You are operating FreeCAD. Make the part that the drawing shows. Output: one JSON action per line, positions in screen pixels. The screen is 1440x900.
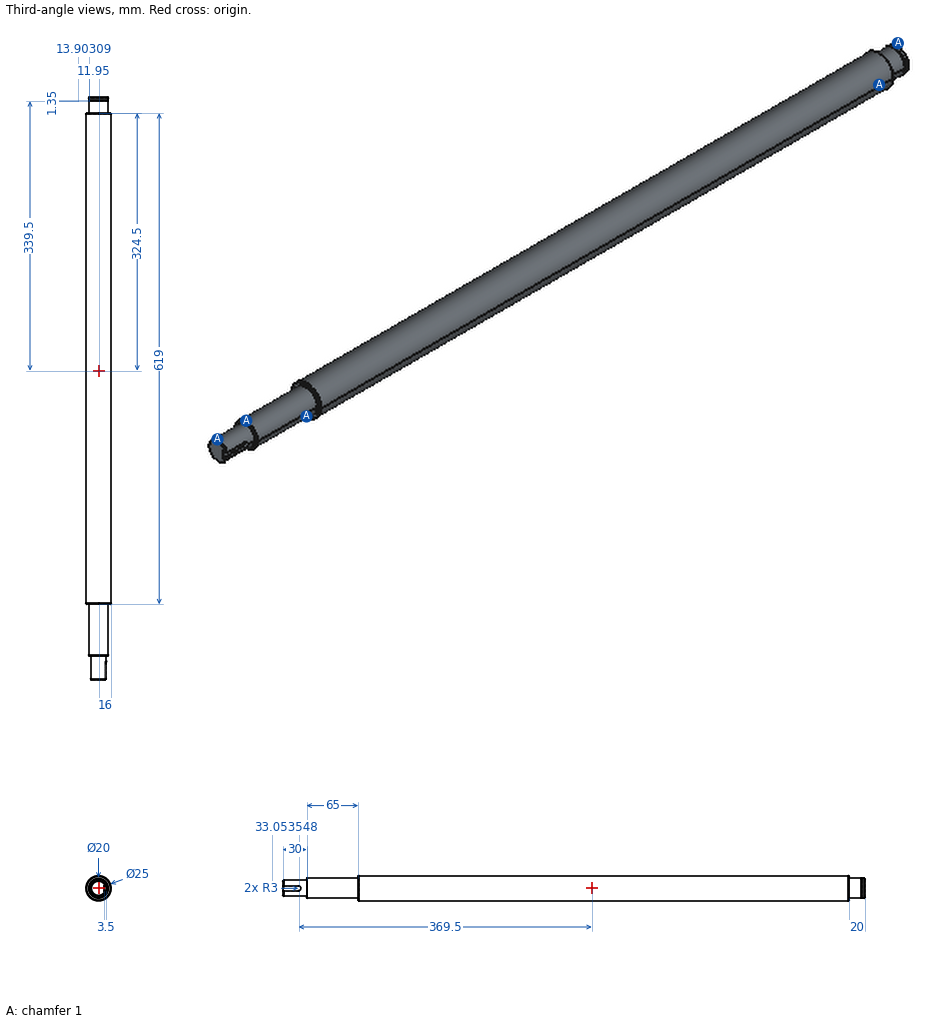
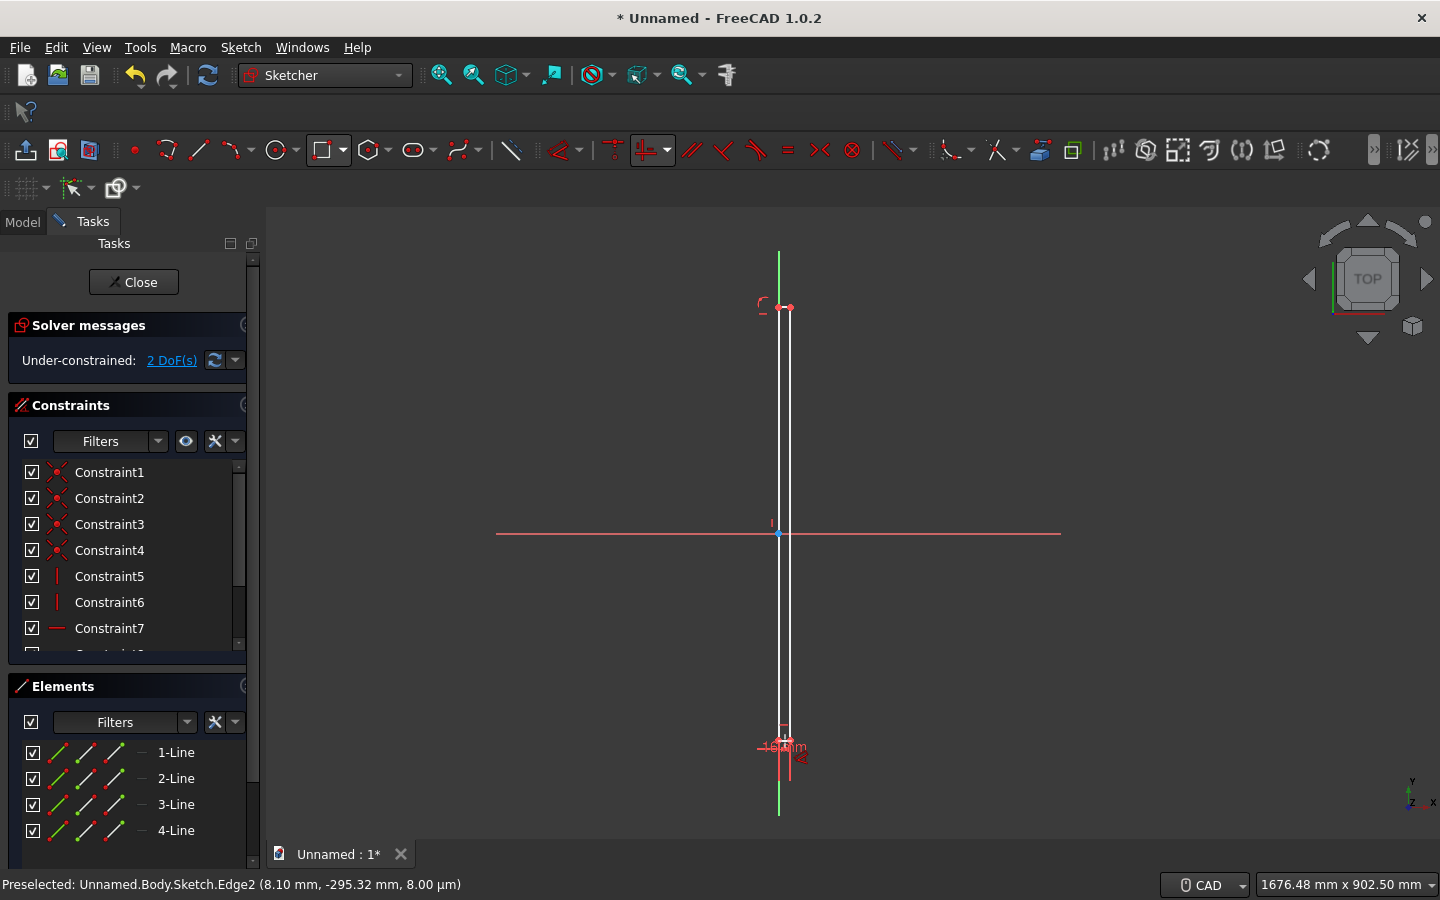
{"action": "scroll", "coordinate": [779, 654], "scroll_direction": "up", "scroll_amount": 2}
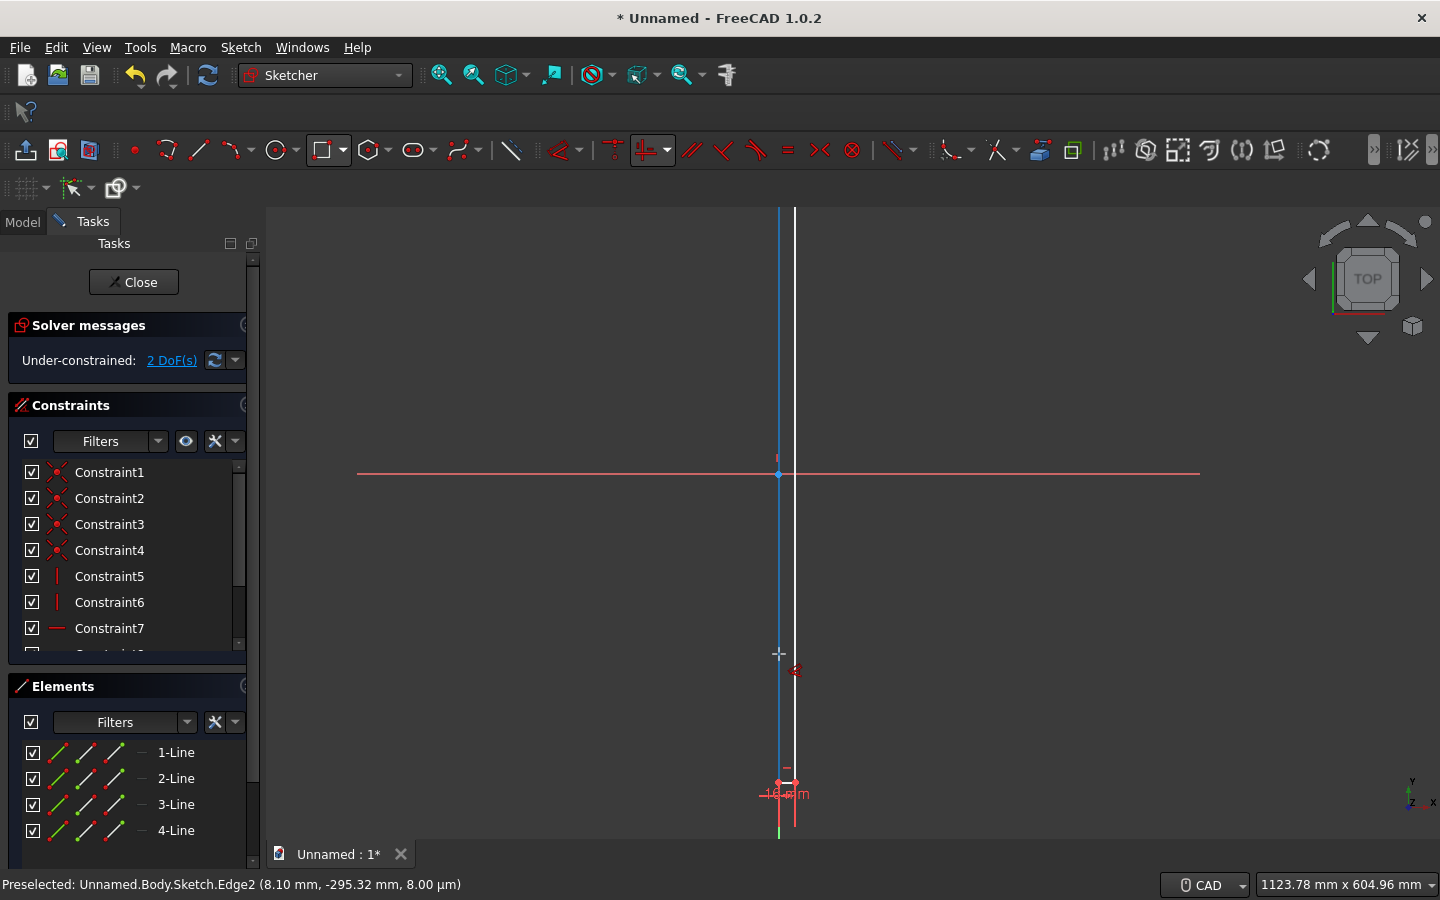
{"action": "left_click", "coordinate": [779, 654]}
{"action": "left_click", "coordinate": [745, 509]}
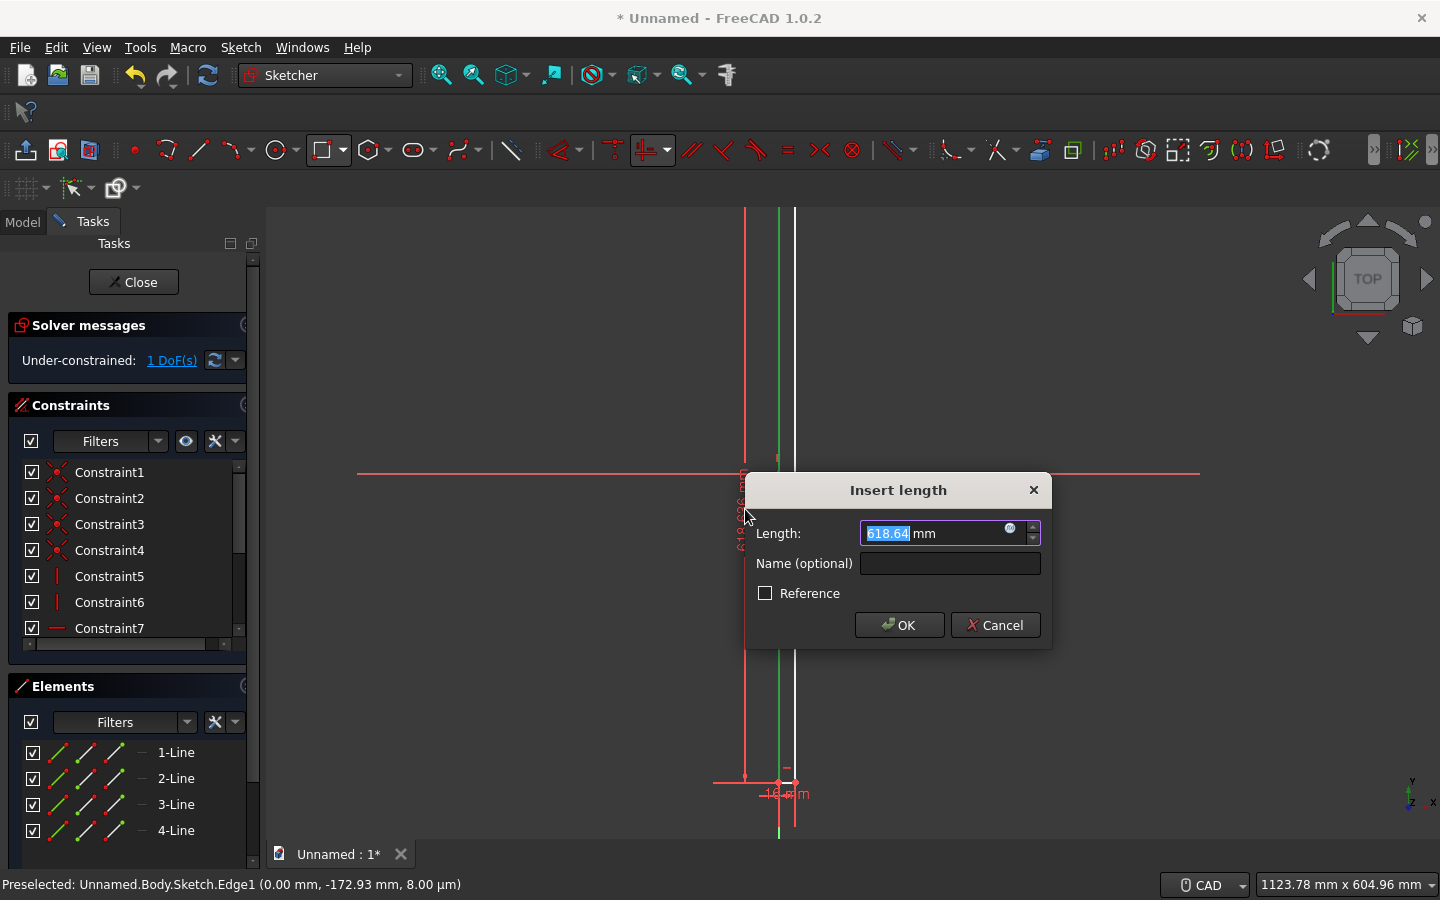
{"action": "type", "text": "619"}
{"action": "key", "text": "Return"}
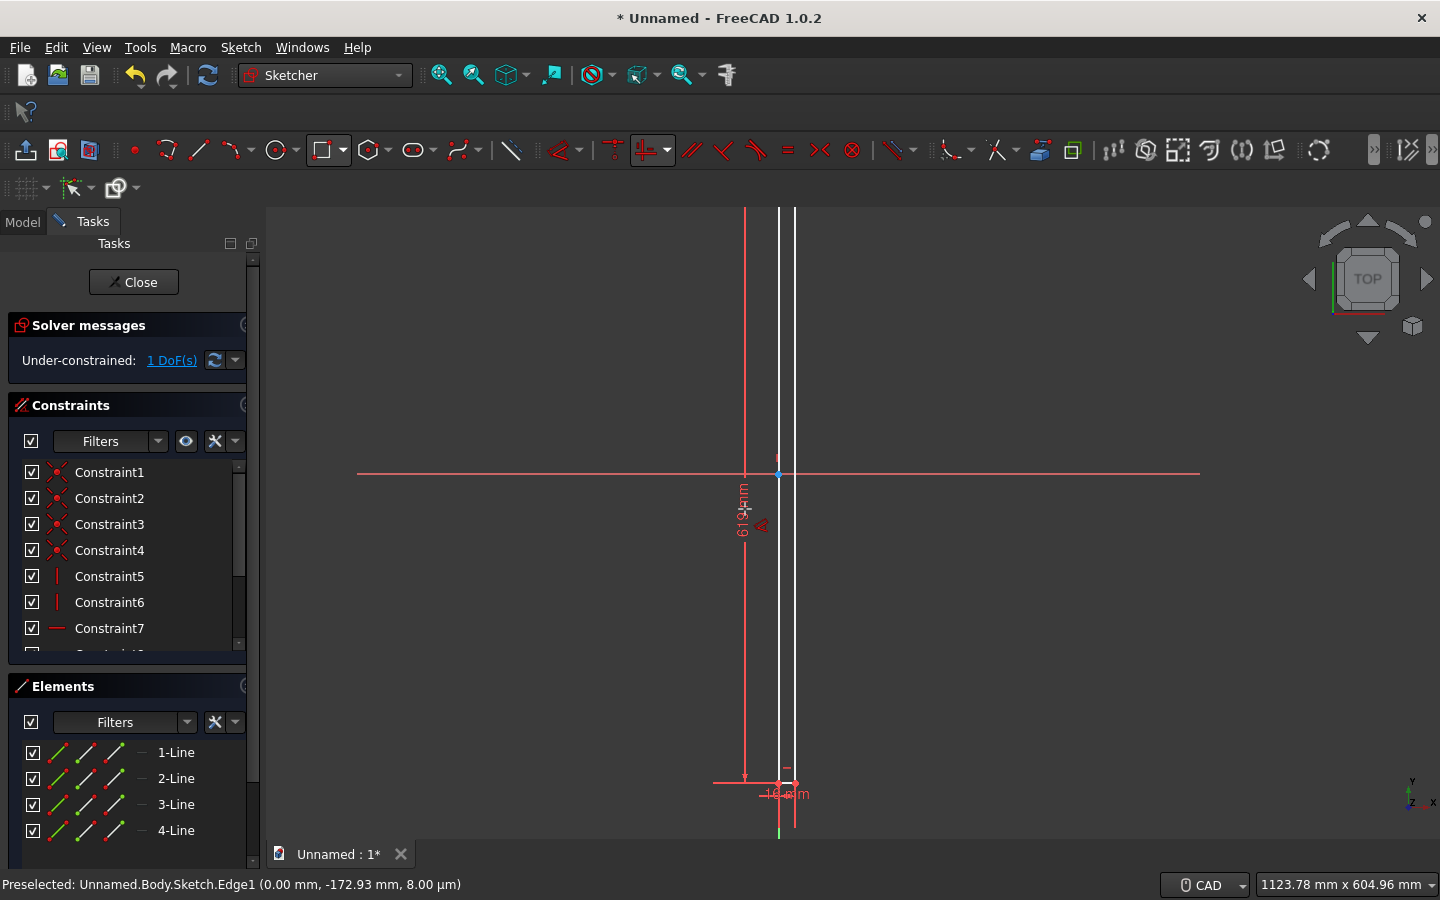
{"action": "scroll", "coordinate": [779, 654], "scroll_direction": "down", "scroll_amount": 2}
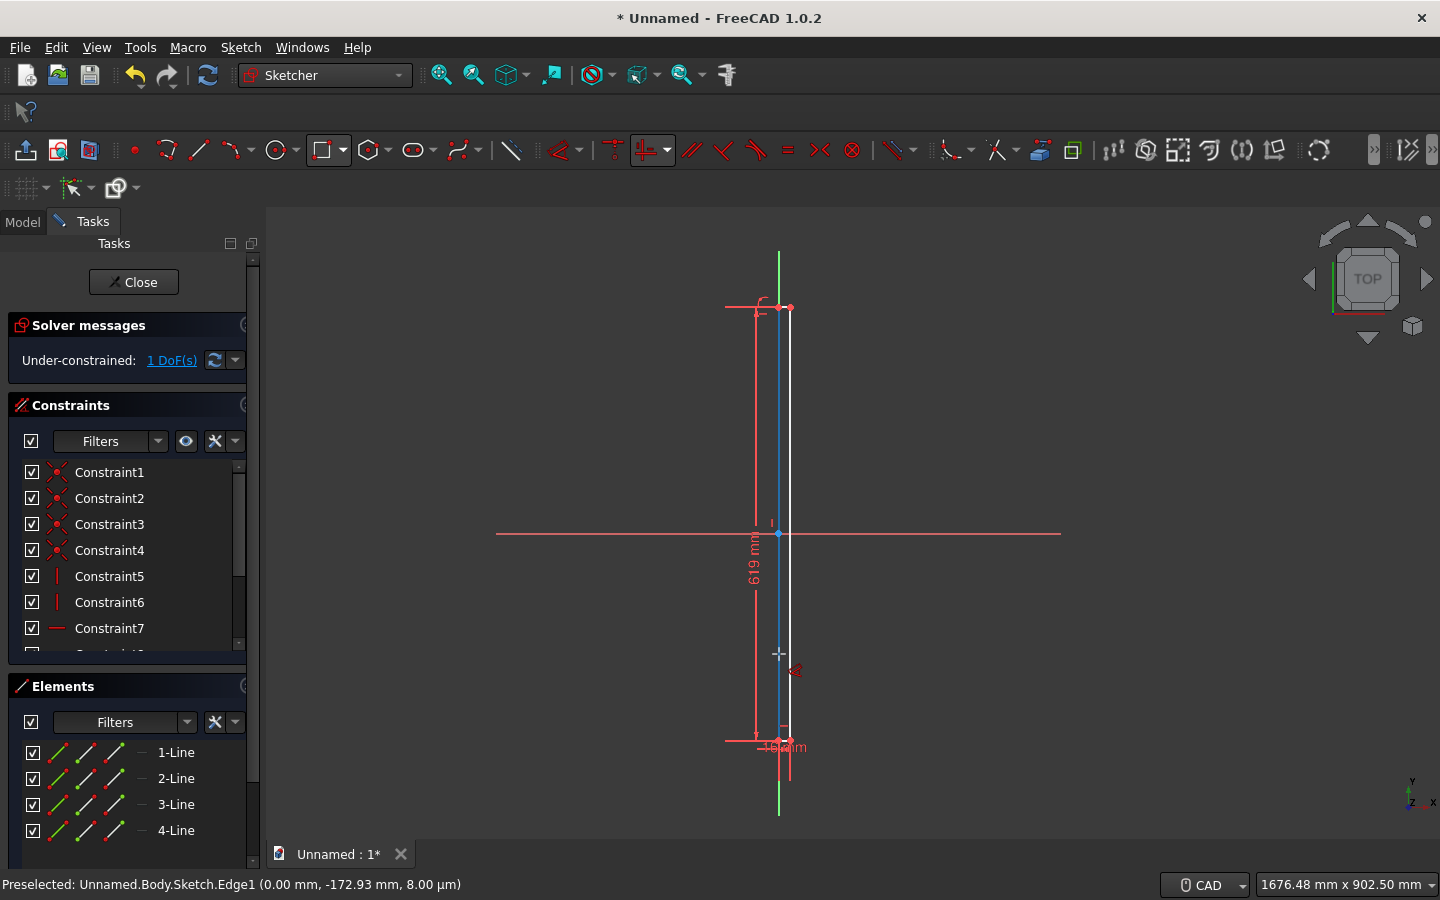
{"action": "left_click", "coordinate": [779, 307]}
{"action": "left_click", "coordinate": [745, 421]}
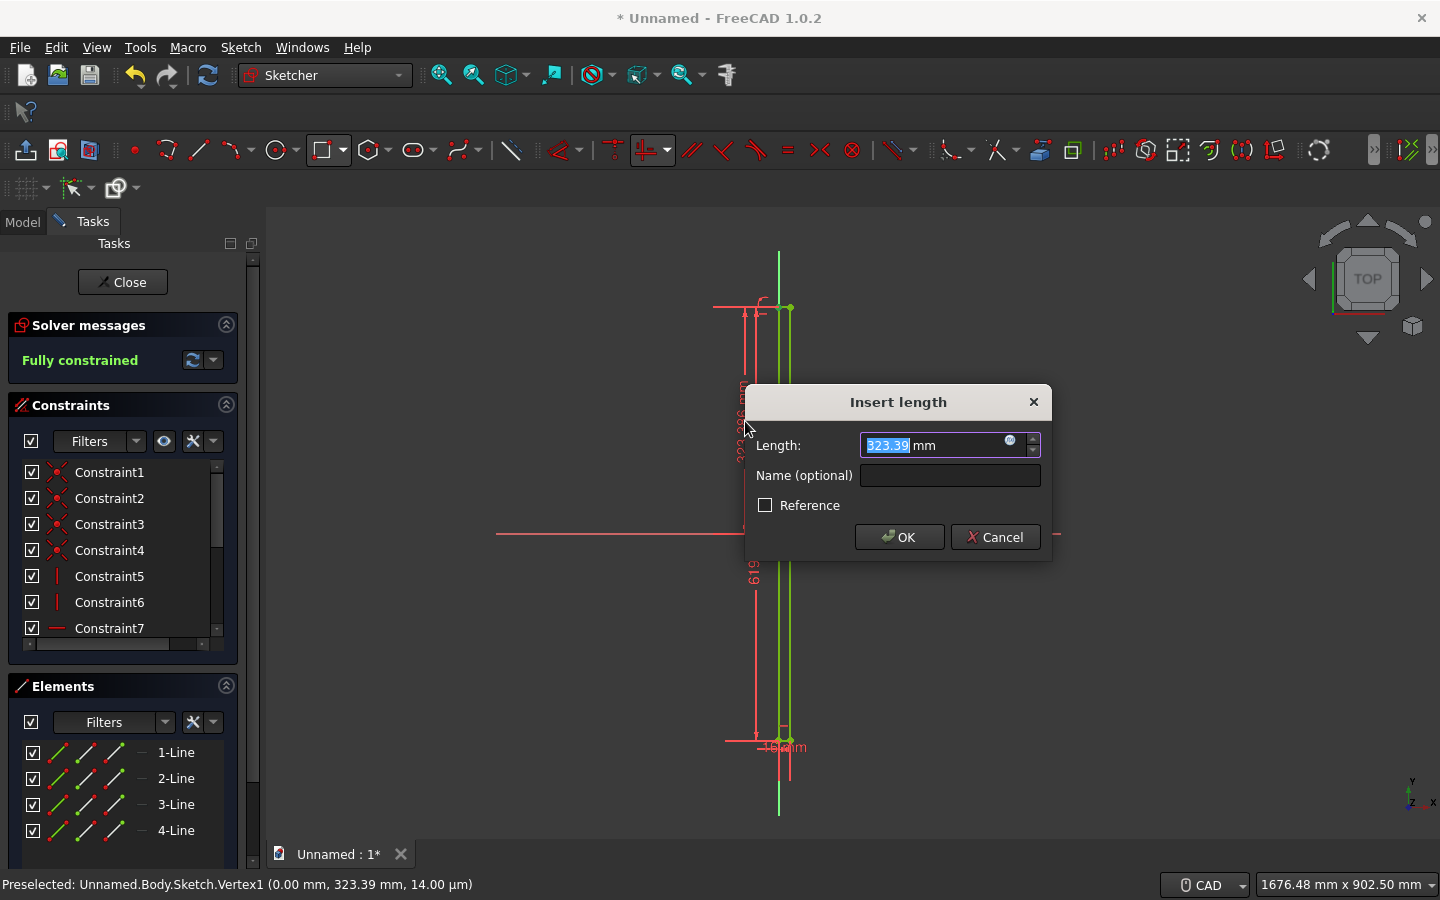
{"action": "type", "text": "324.5"}
{"action": "key", "text": "Return"}
{"action": "key", "text": "Escape"}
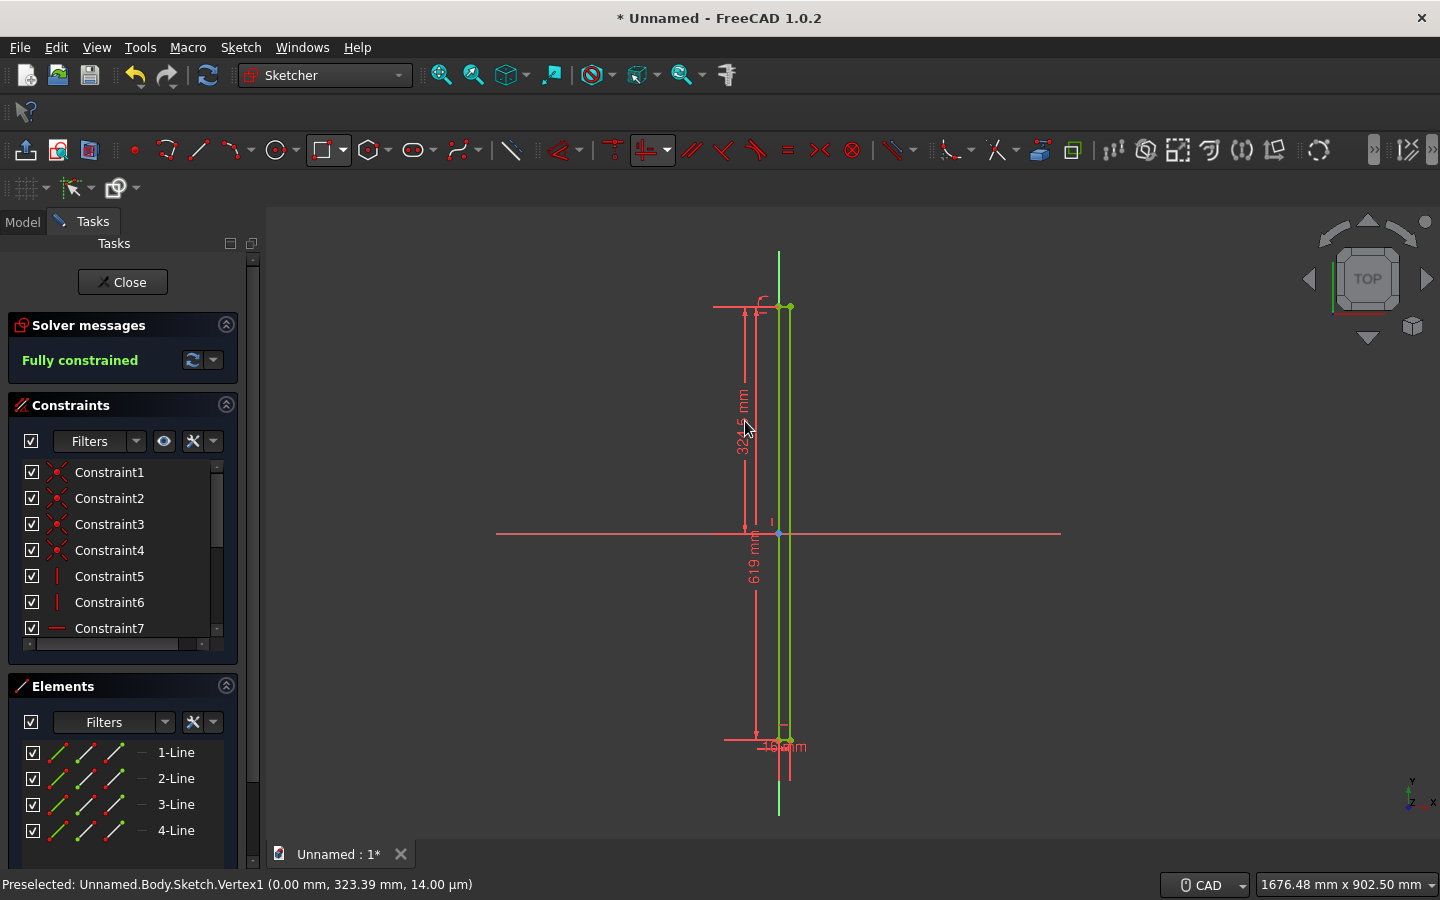
{"action": "left_click", "coordinate": [123, 282]}